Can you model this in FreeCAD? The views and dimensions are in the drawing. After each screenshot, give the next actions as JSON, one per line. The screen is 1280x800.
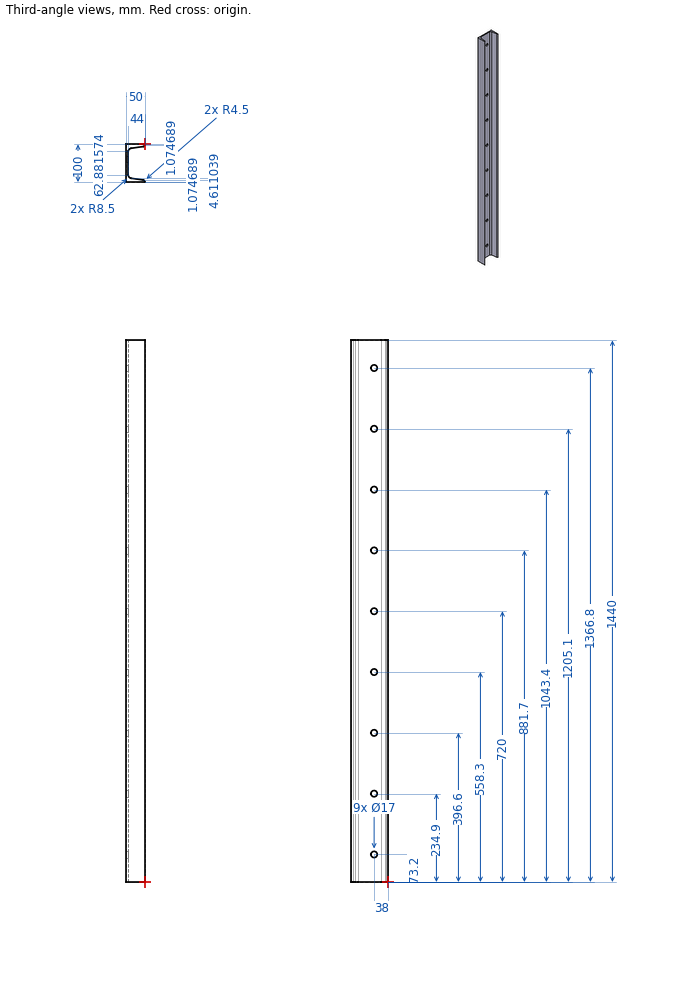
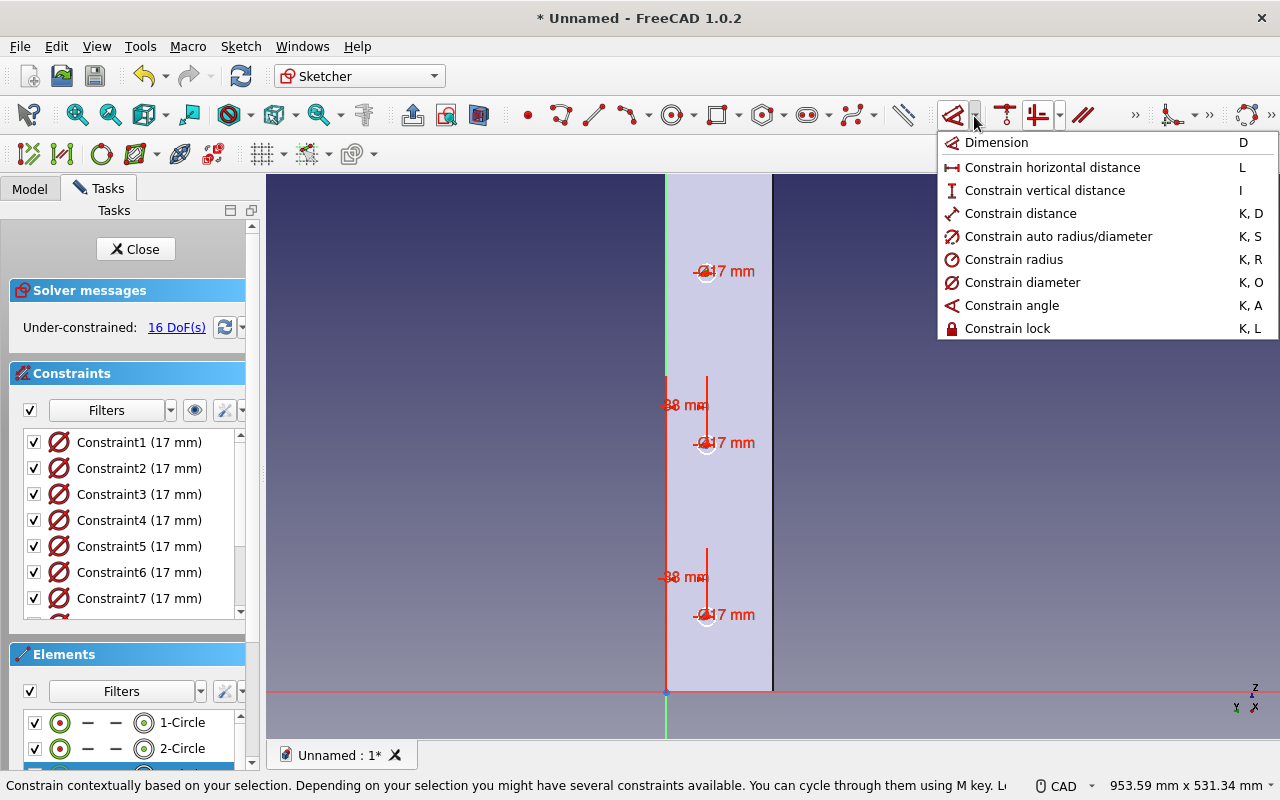
{"action": "left_click", "coordinate": [1108, 168]}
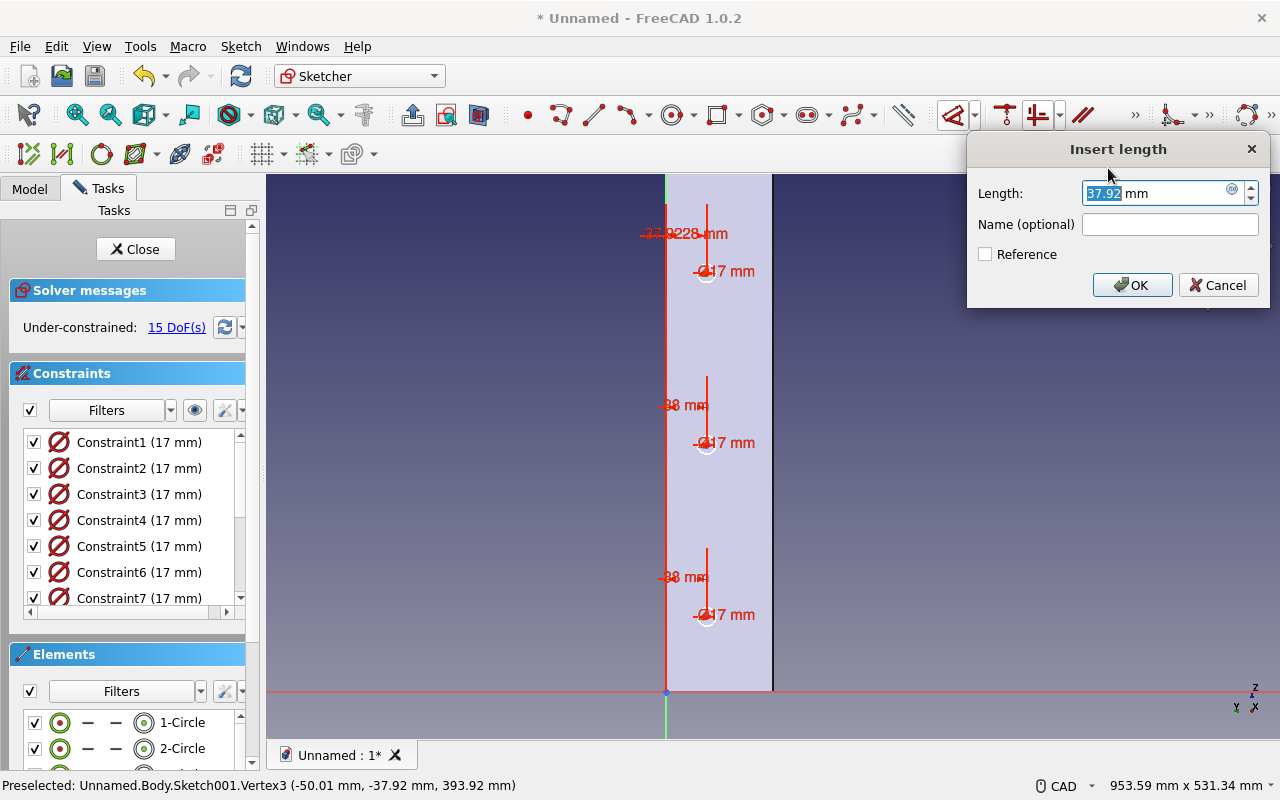
{"action": "type", "text": "38"}
{"action": "key", "text": "Return"}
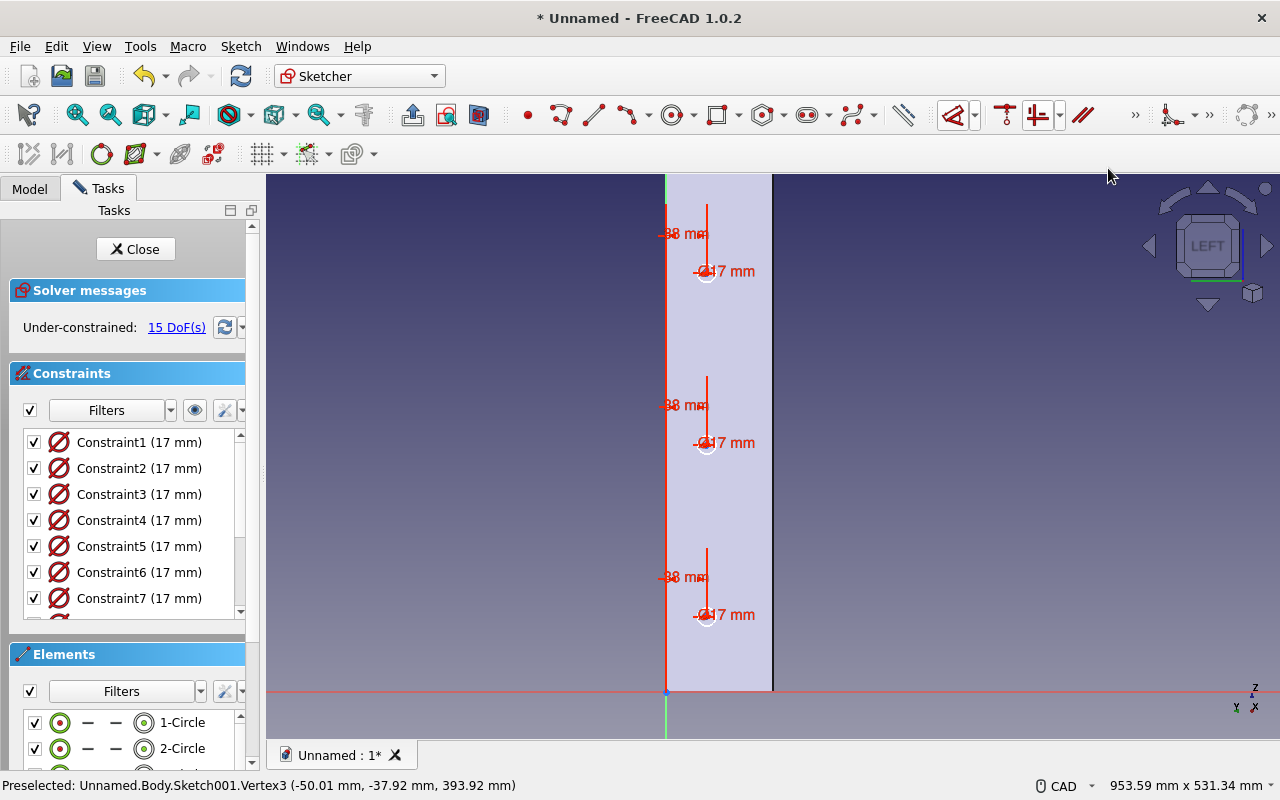
{"action": "scroll", "coordinate": [709, 619], "scroll_direction": "down", "scroll_amount": 7}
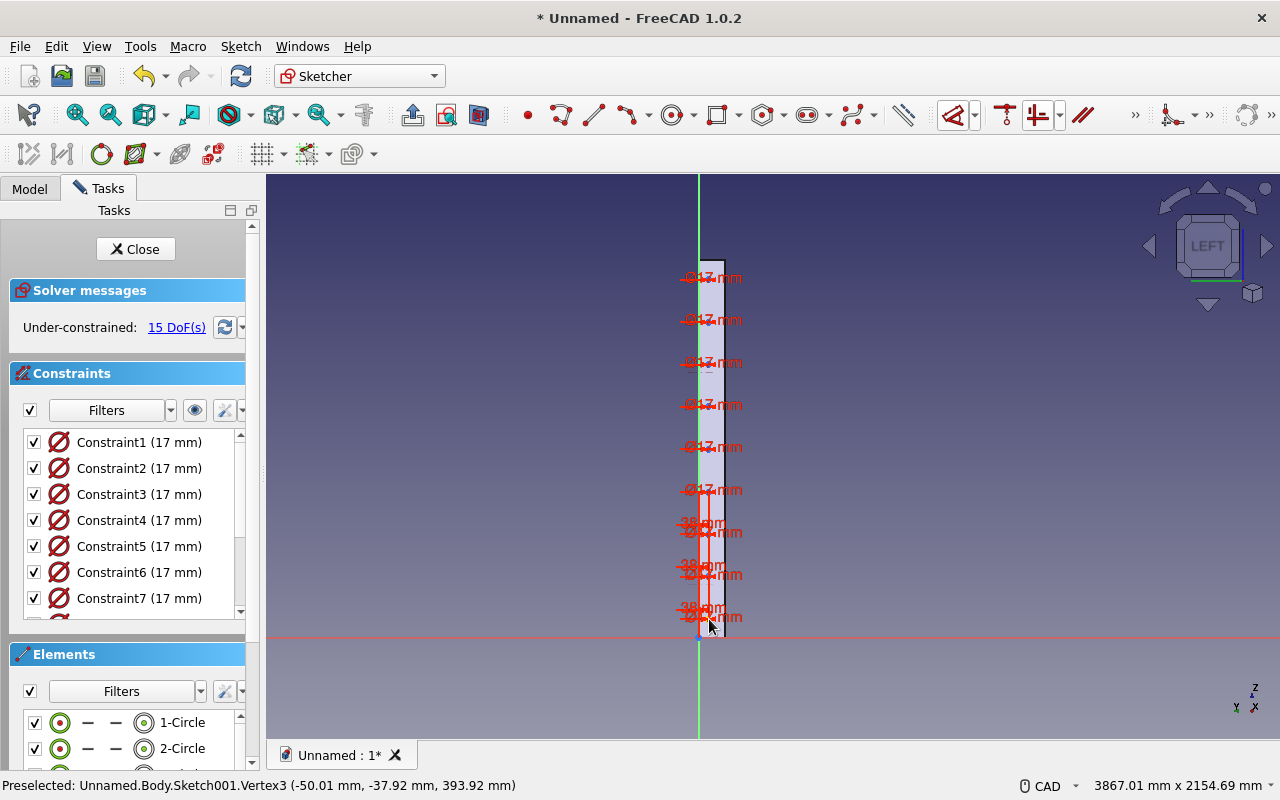
{"action": "scroll", "coordinate": [709, 492], "scroll_direction": "up", "scroll_amount": 7}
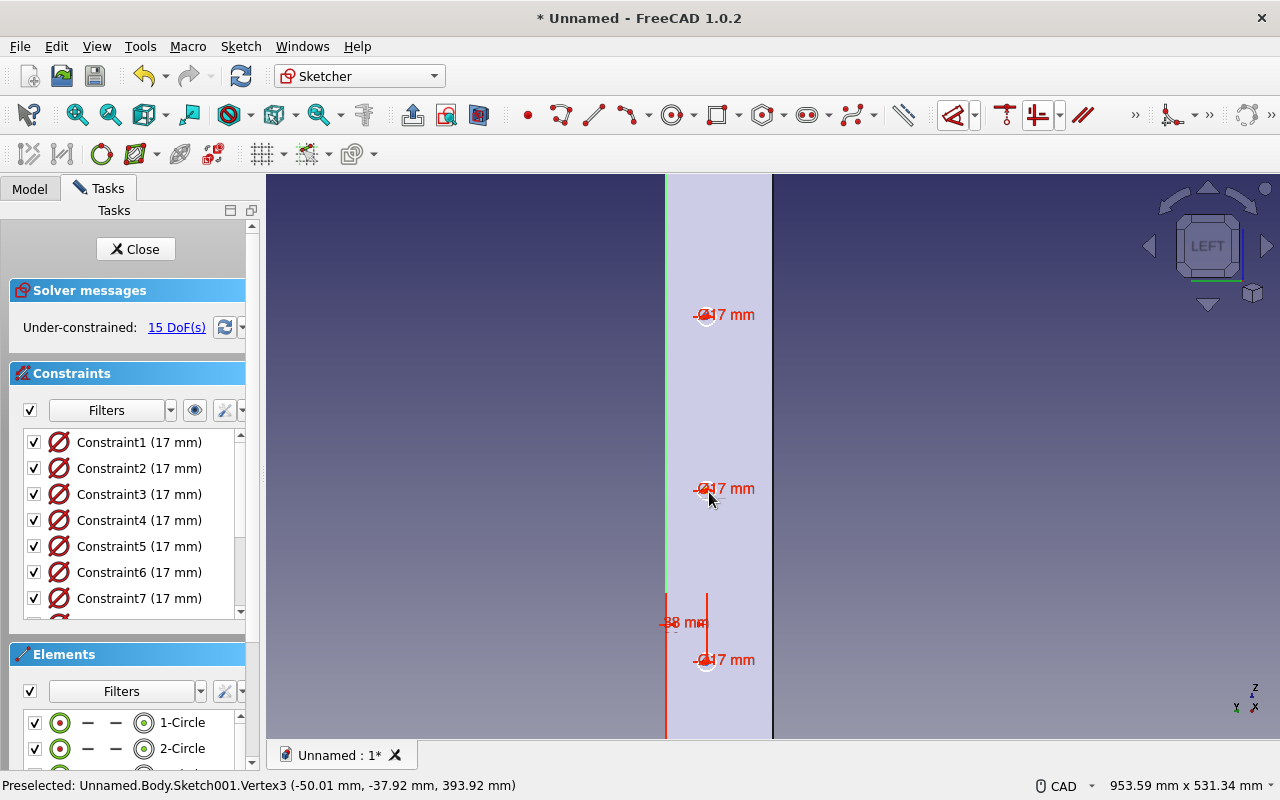
{"action": "left_click", "coordinate": [707, 491]}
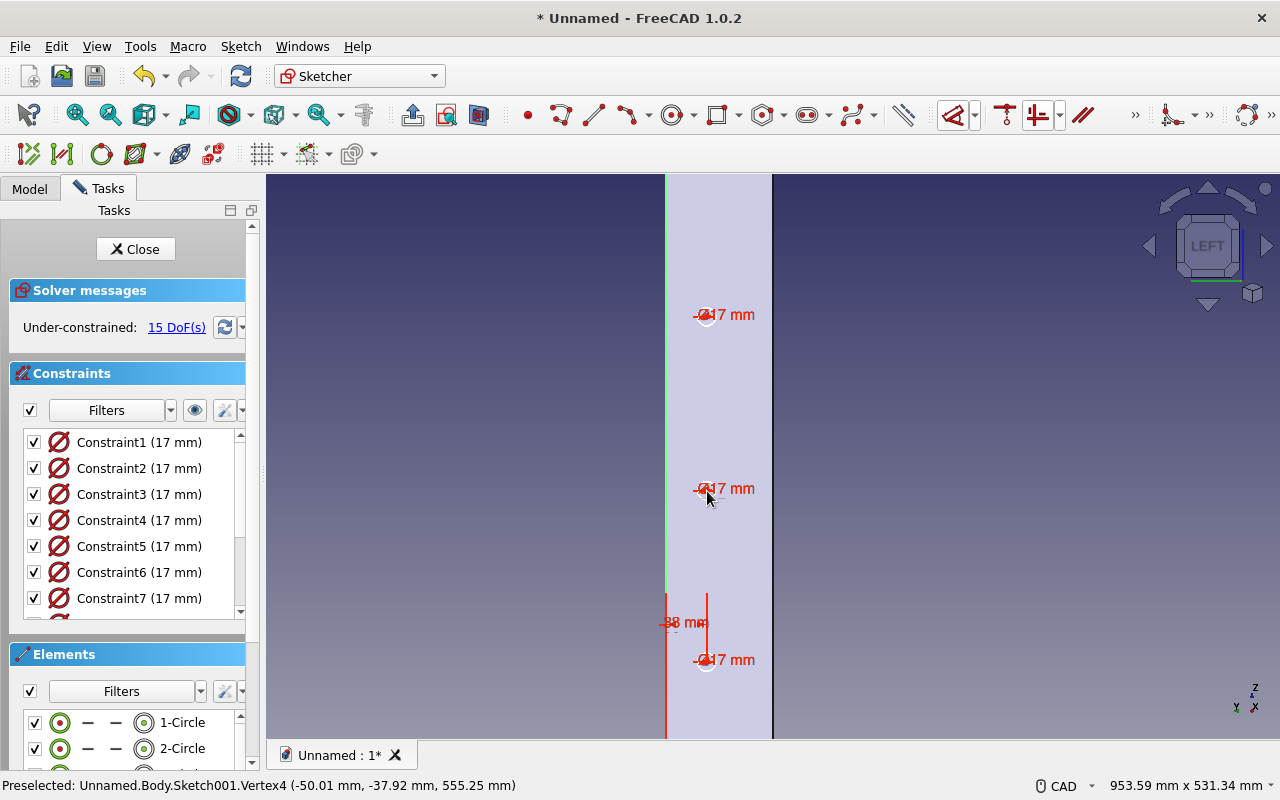
{"action": "left_click", "coordinate": [974, 116]}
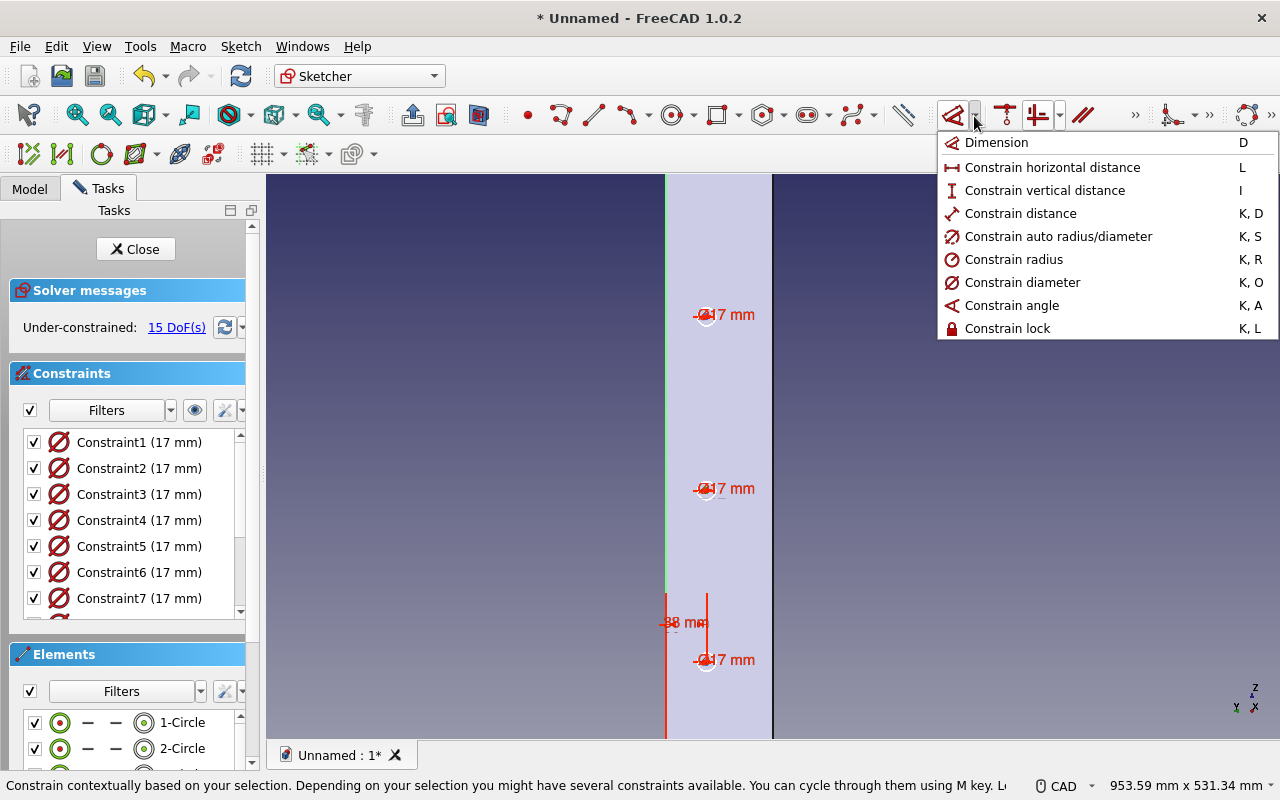
{"action": "left_click", "coordinate": [1108, 168]}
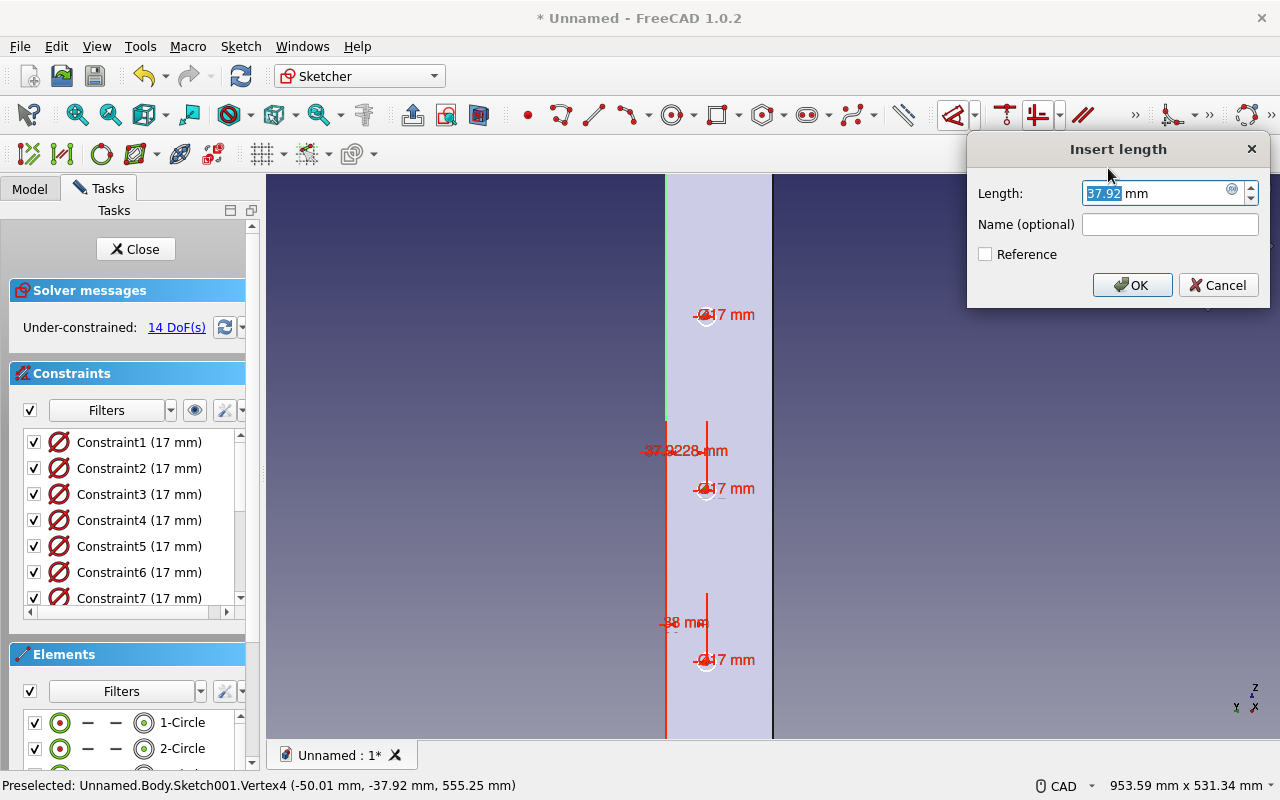
{"action": "type", "text": "38"}
{"action": "key", "text": "Return"}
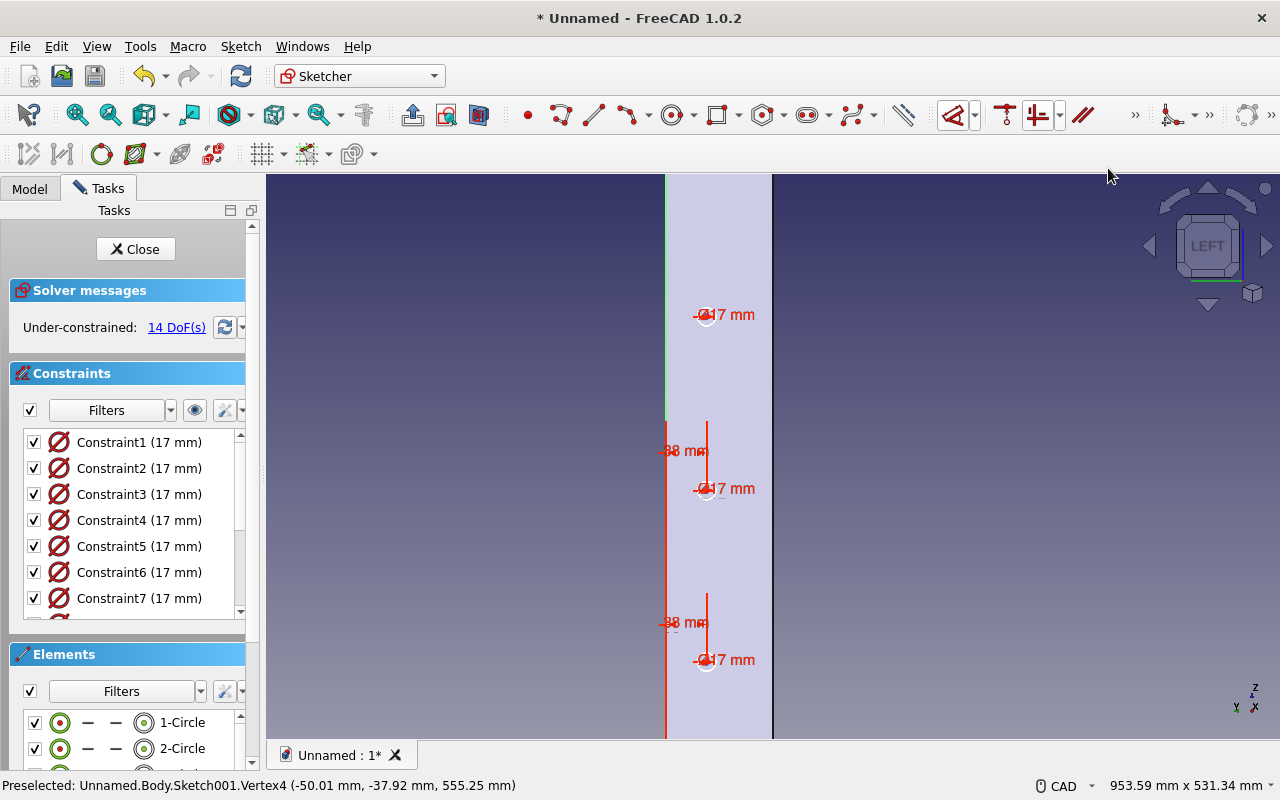
{"action": "left_click", "coordinate": [707, 317]}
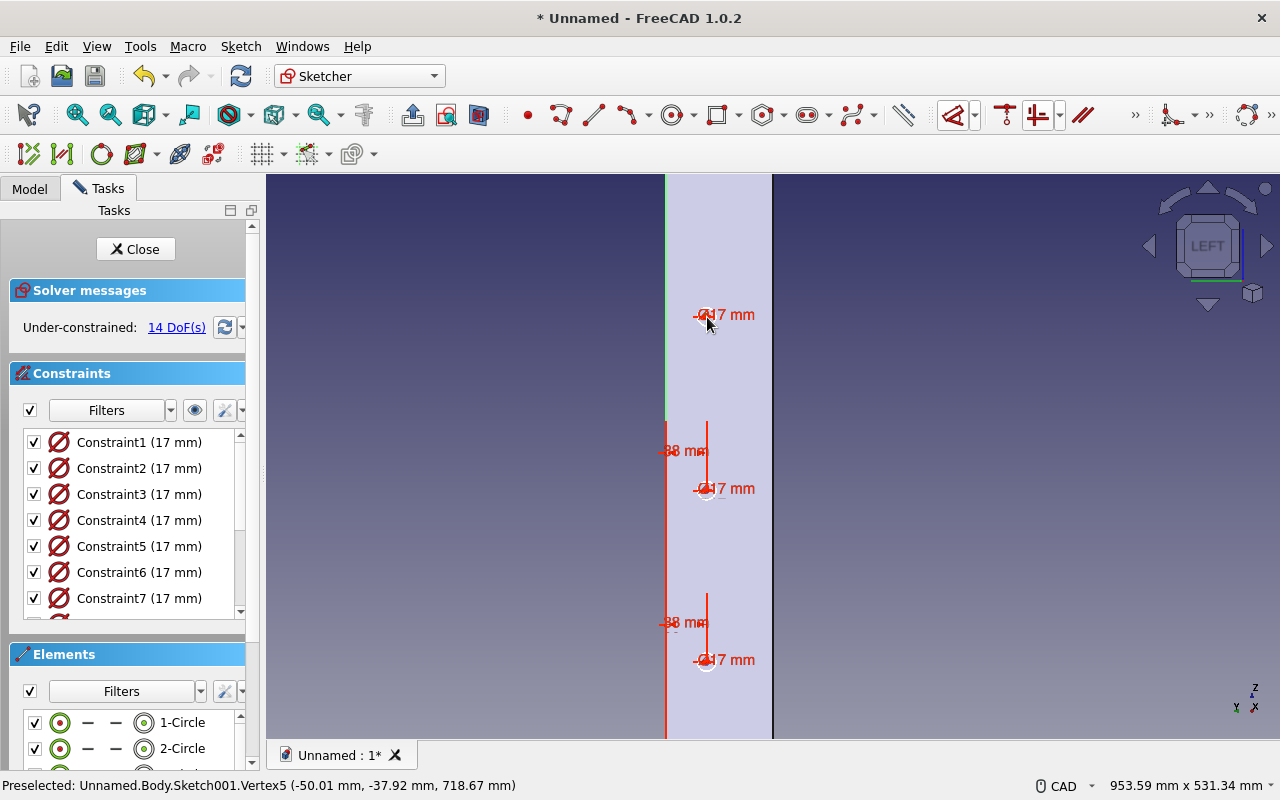
{"action": "left_click", "coordinate": [974, 116]}